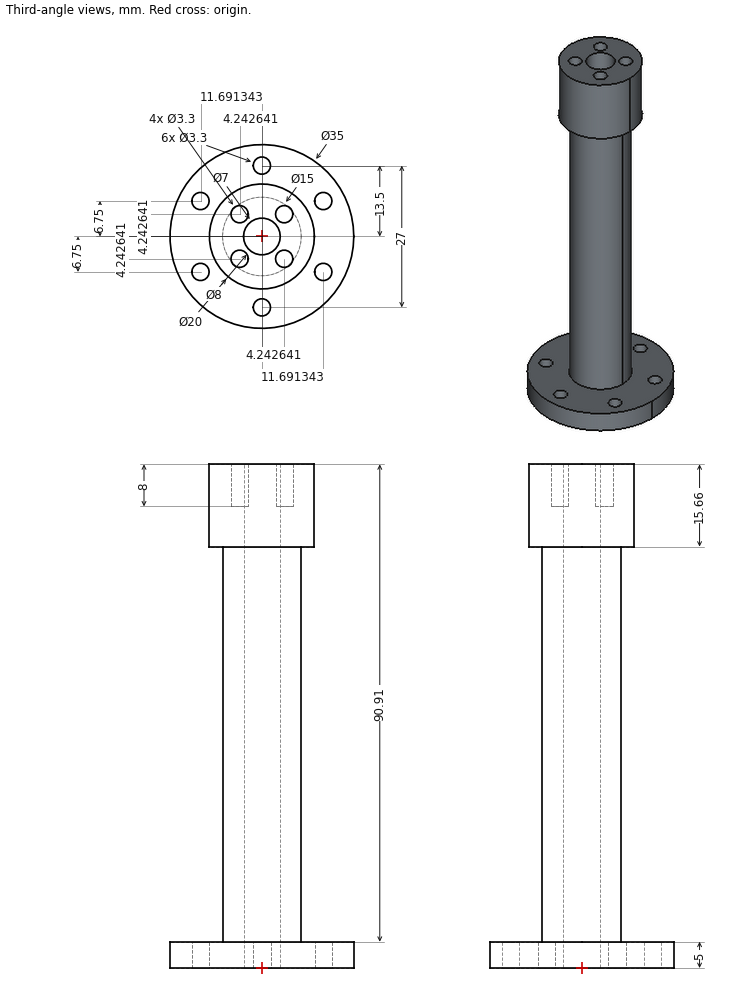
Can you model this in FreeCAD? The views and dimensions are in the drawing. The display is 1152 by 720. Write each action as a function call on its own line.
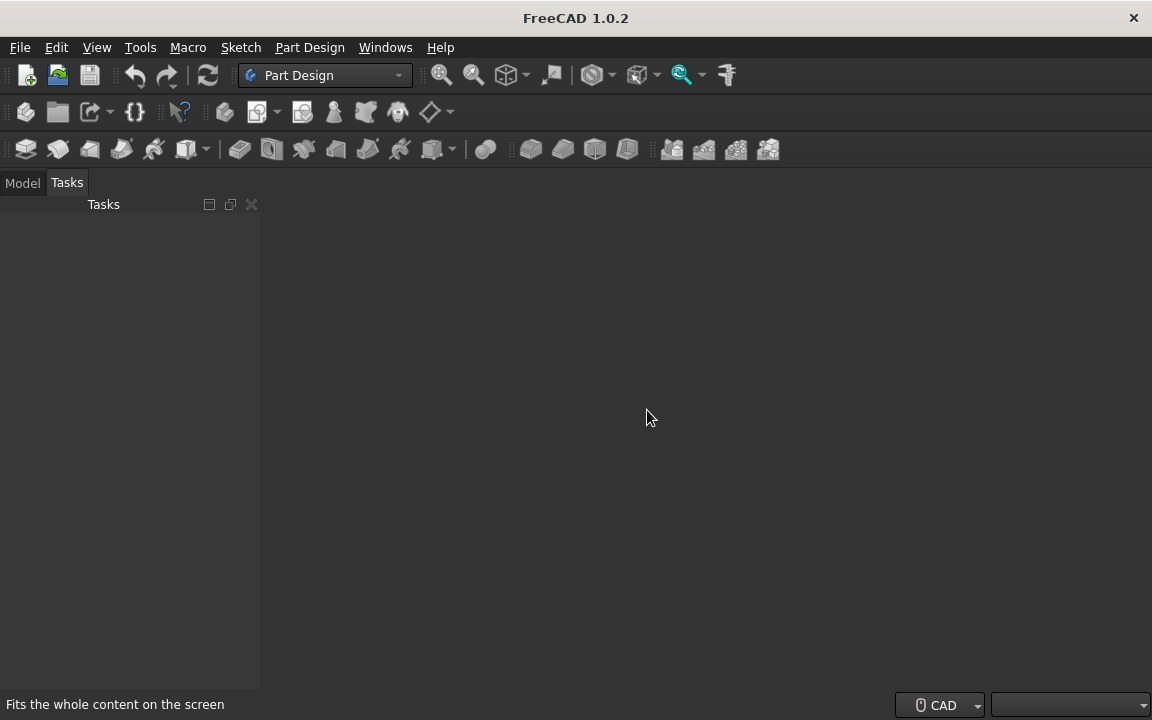
key(ctrl+n)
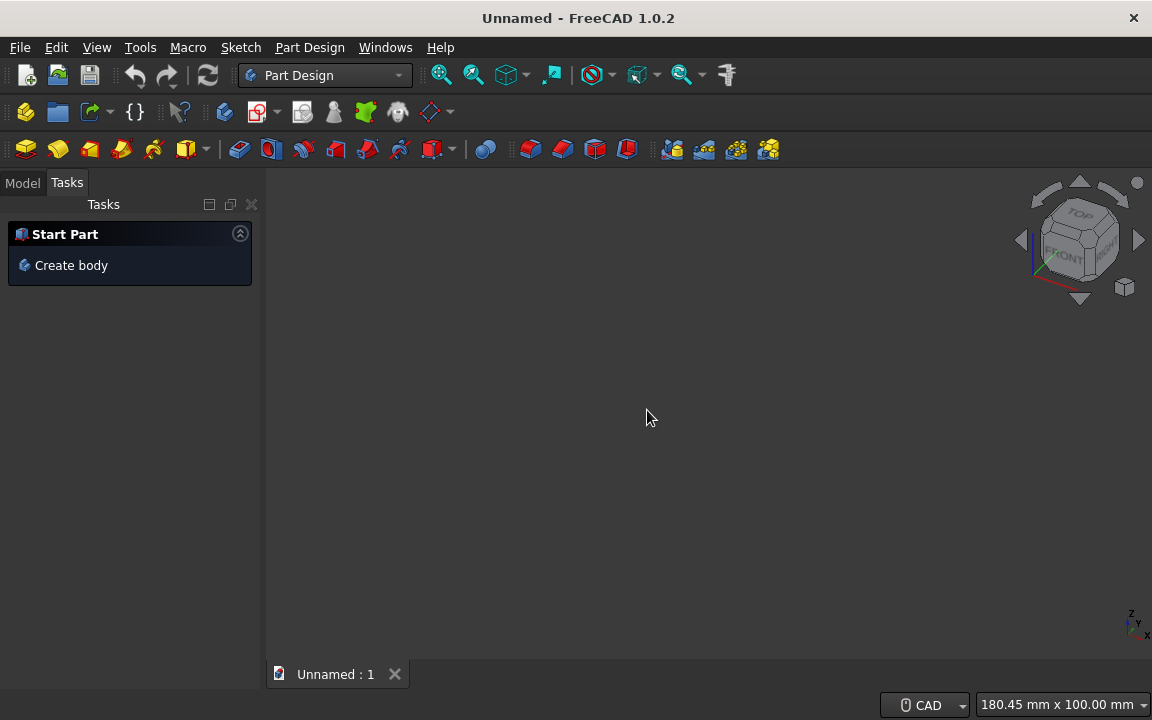
click(258, 112)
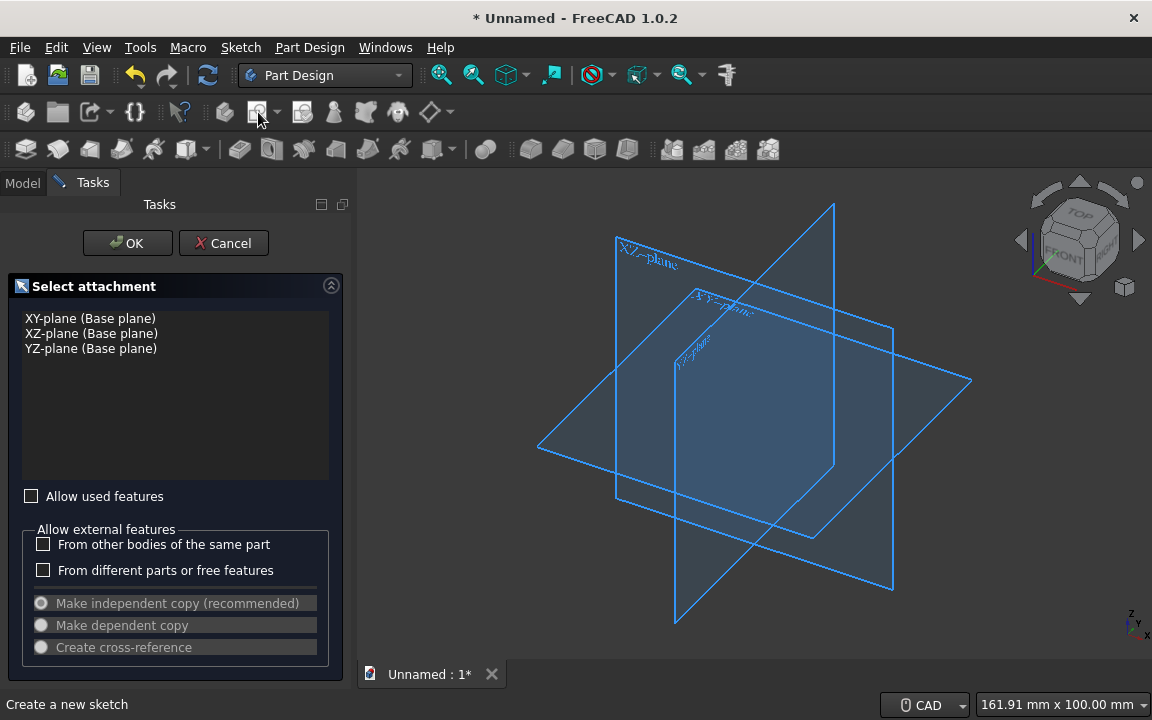
click(82, 318)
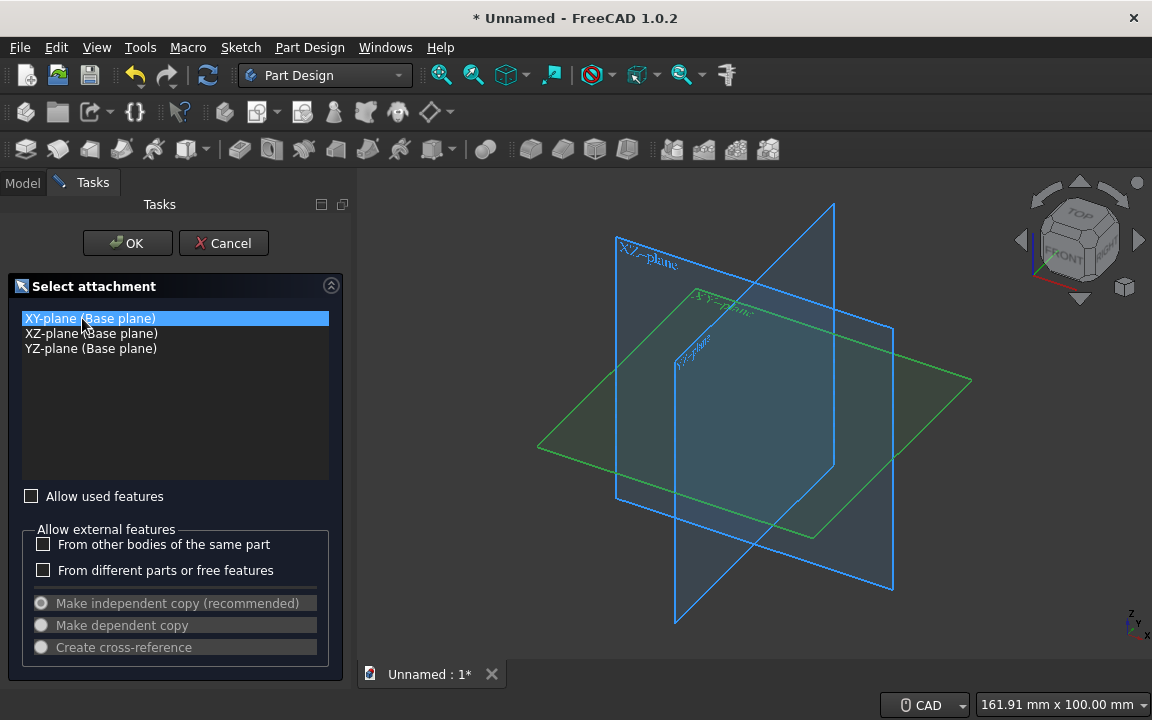
click(128, 243)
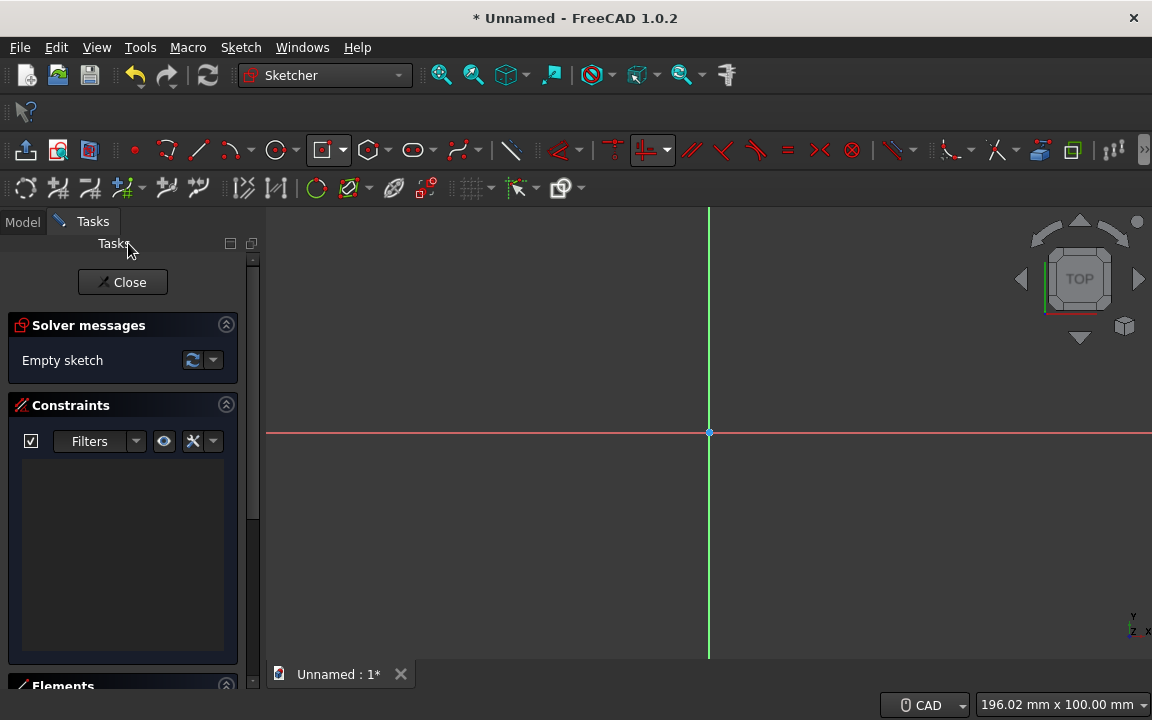
scroll(792, 433, up, 3)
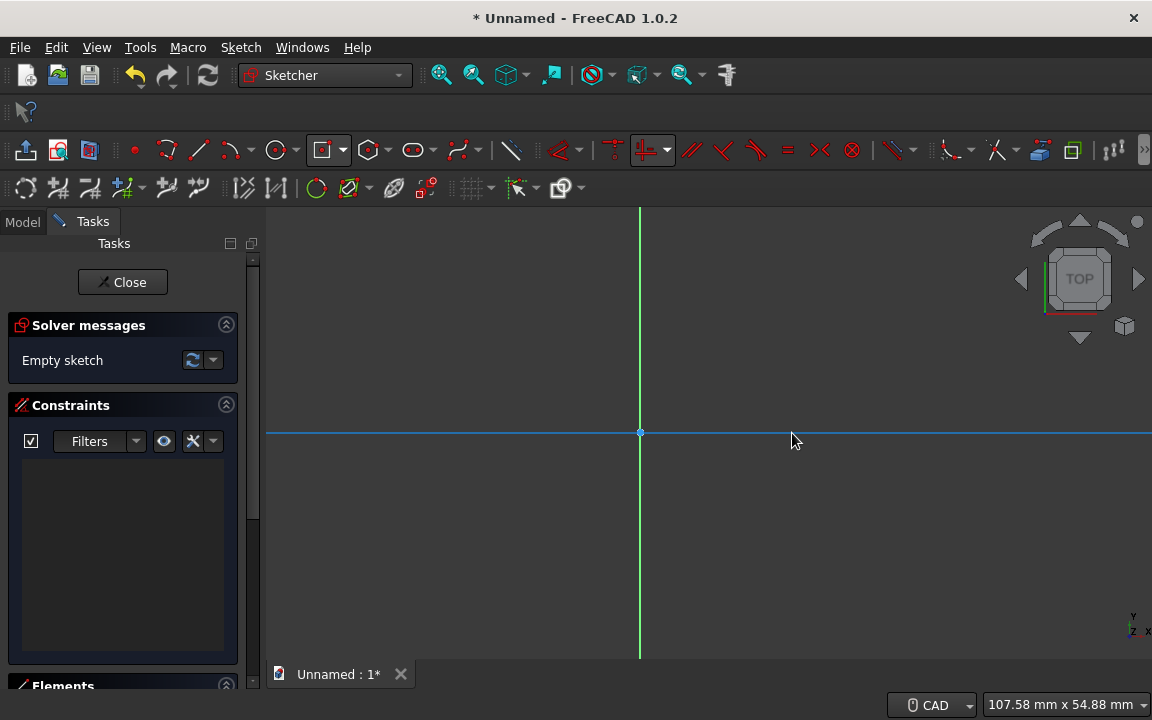
key(g)
key(c)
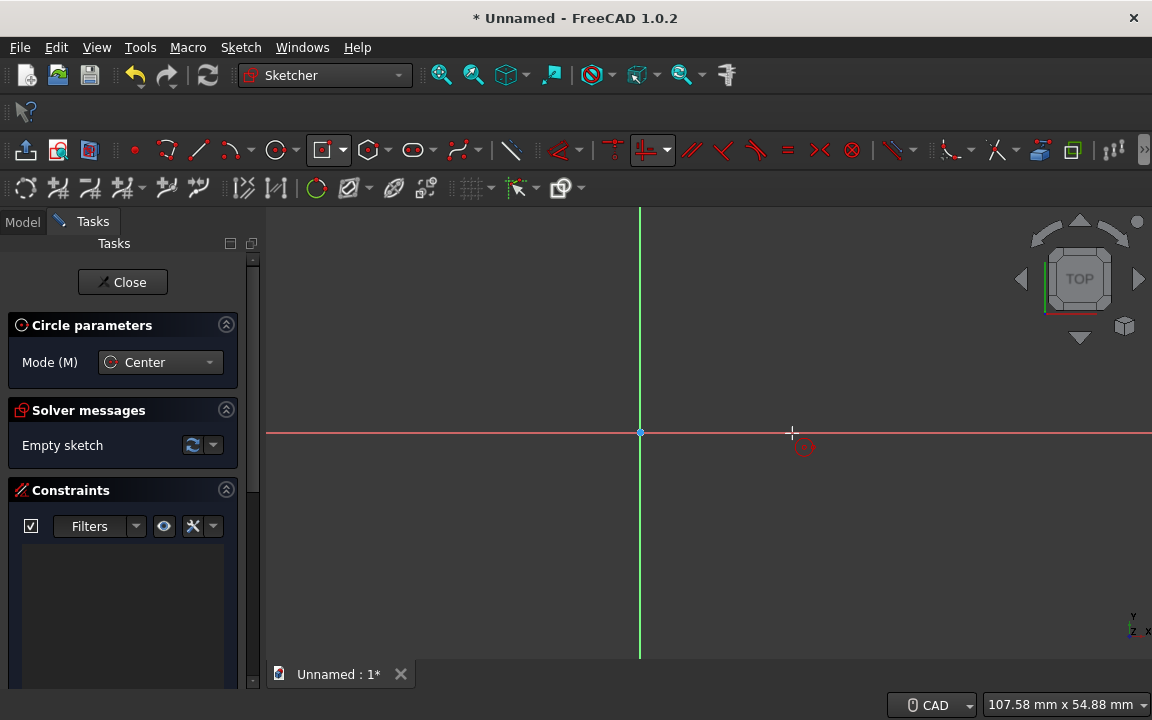
click(640, 433)
click(742, 331)
key(Escape)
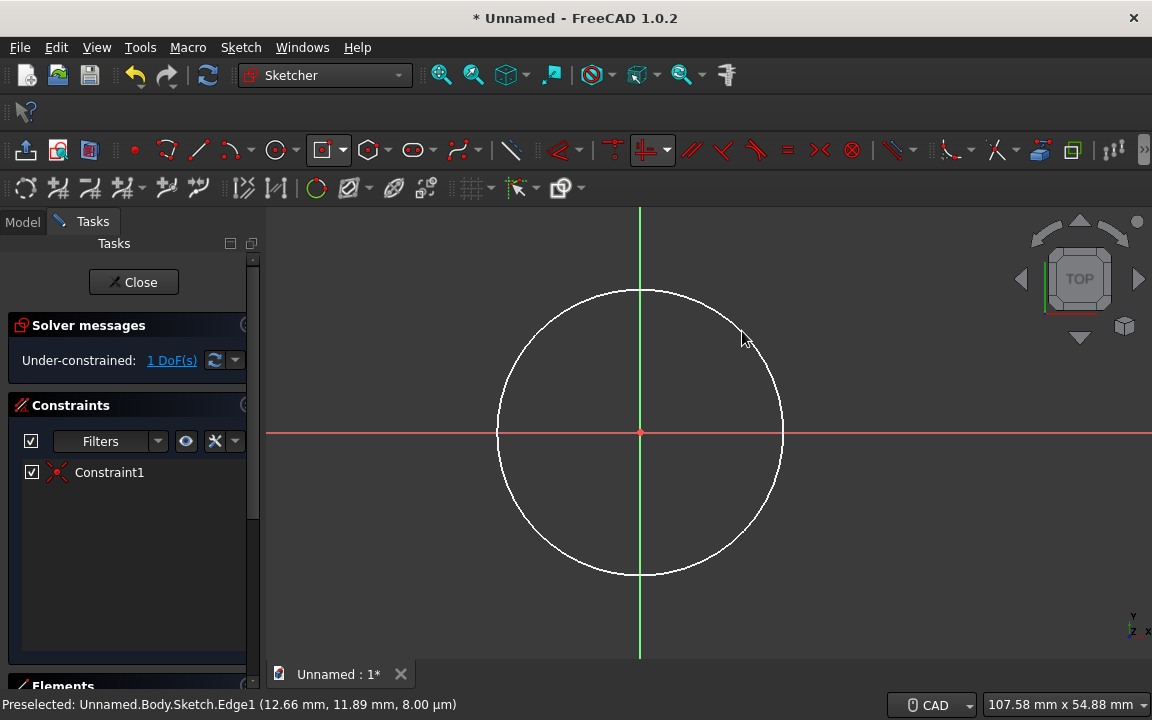
key(d)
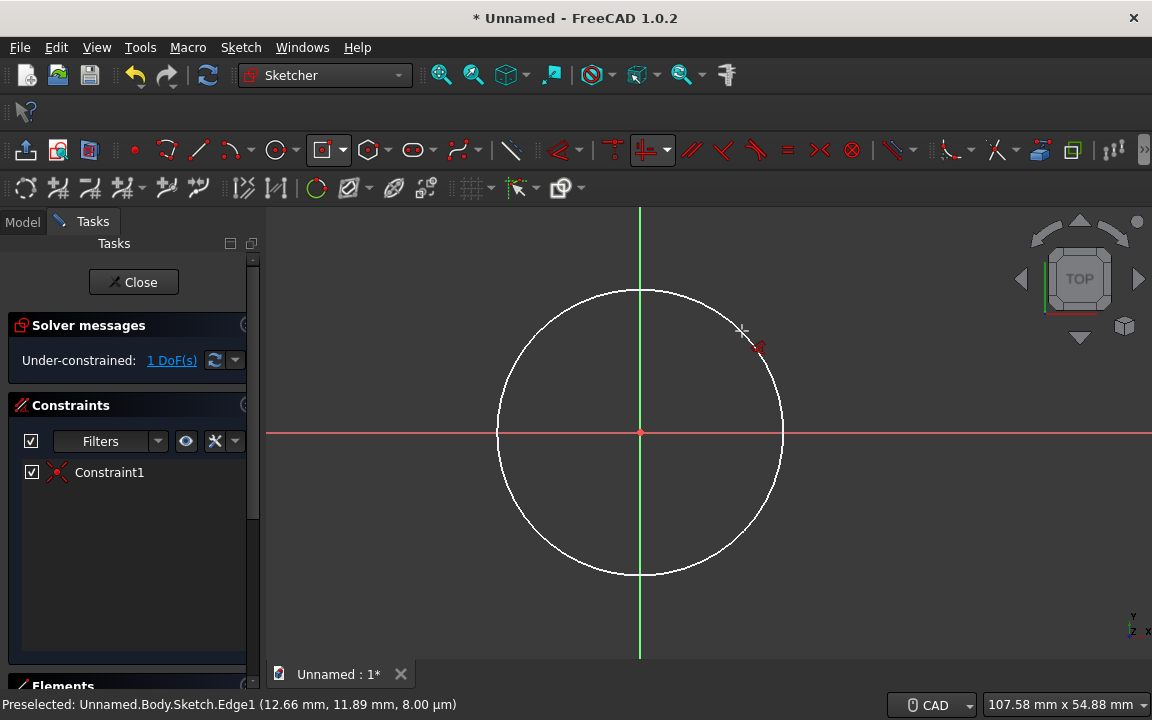
click(741, 331)
click(764, 308)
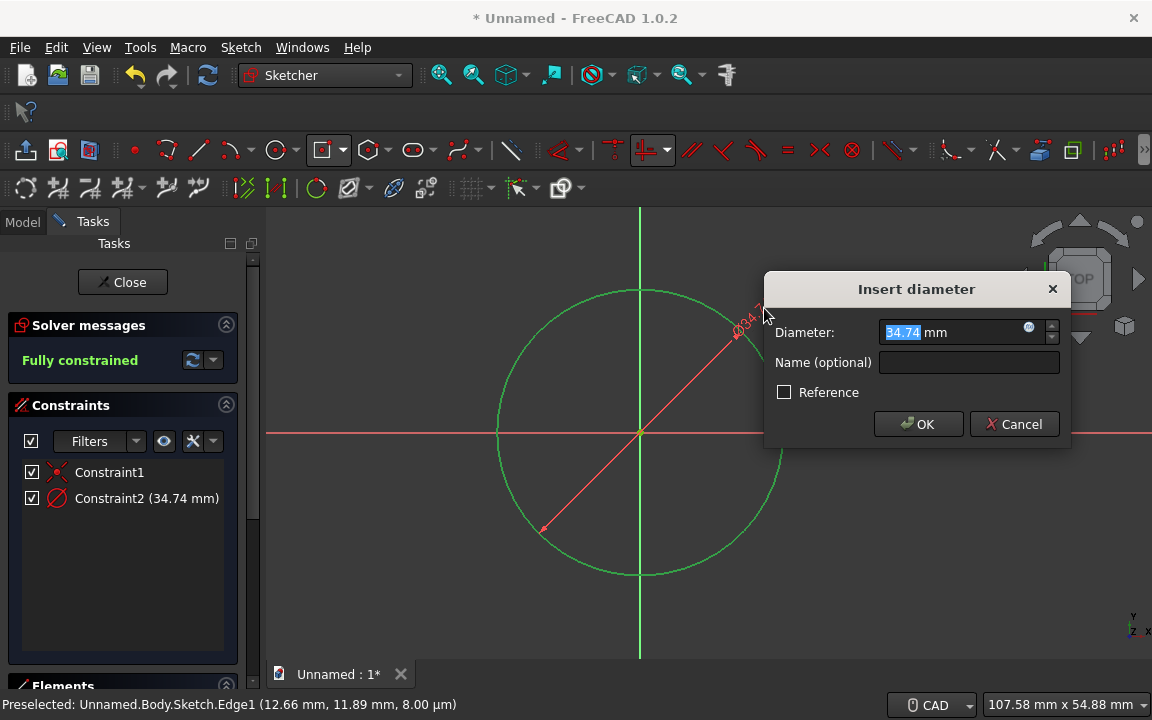
text(35)
key(Return)
key(Escape)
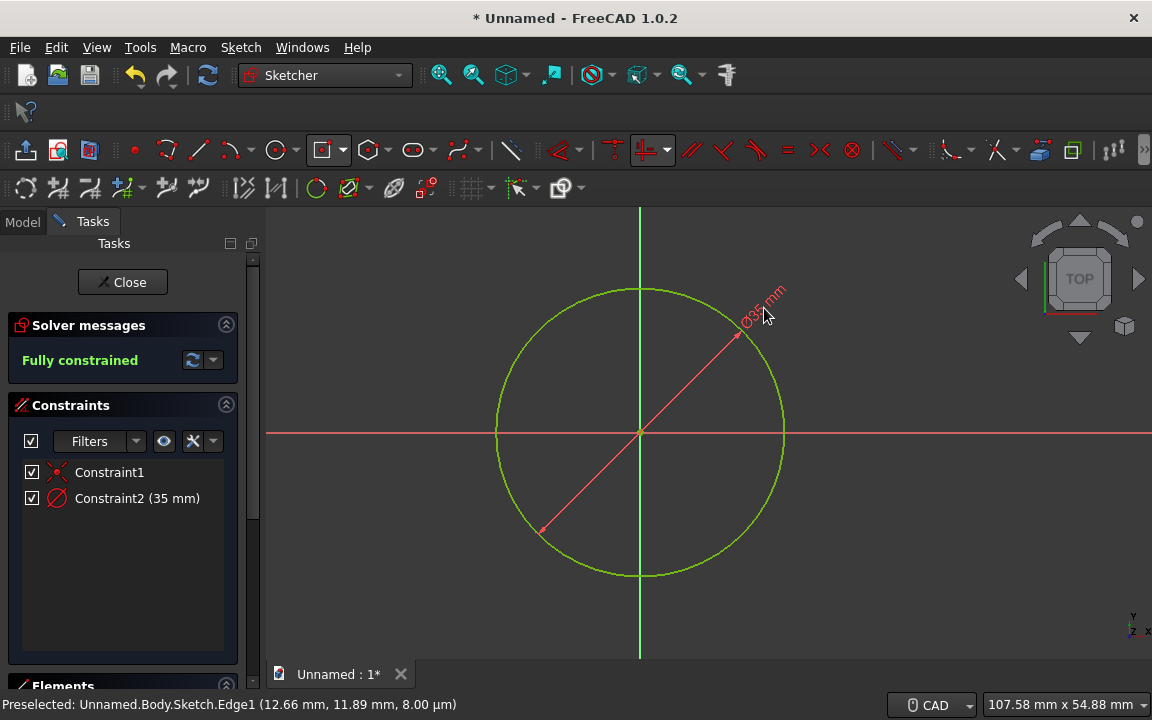
click(123, 282)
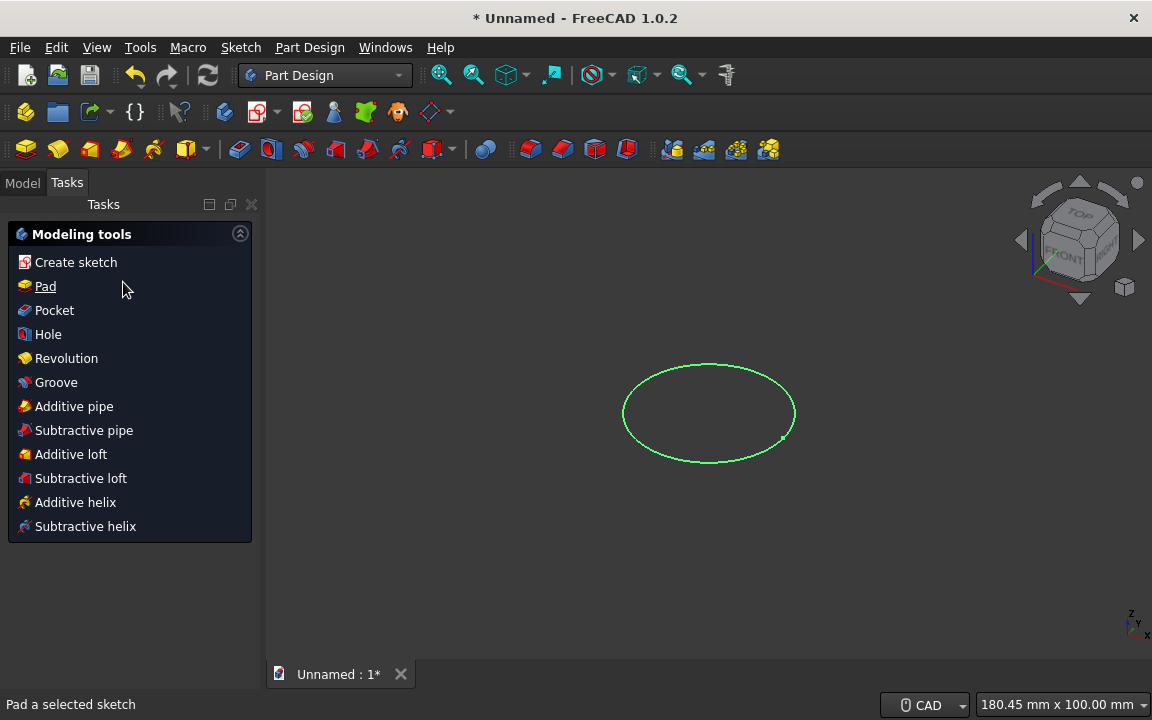
click(26, 150)